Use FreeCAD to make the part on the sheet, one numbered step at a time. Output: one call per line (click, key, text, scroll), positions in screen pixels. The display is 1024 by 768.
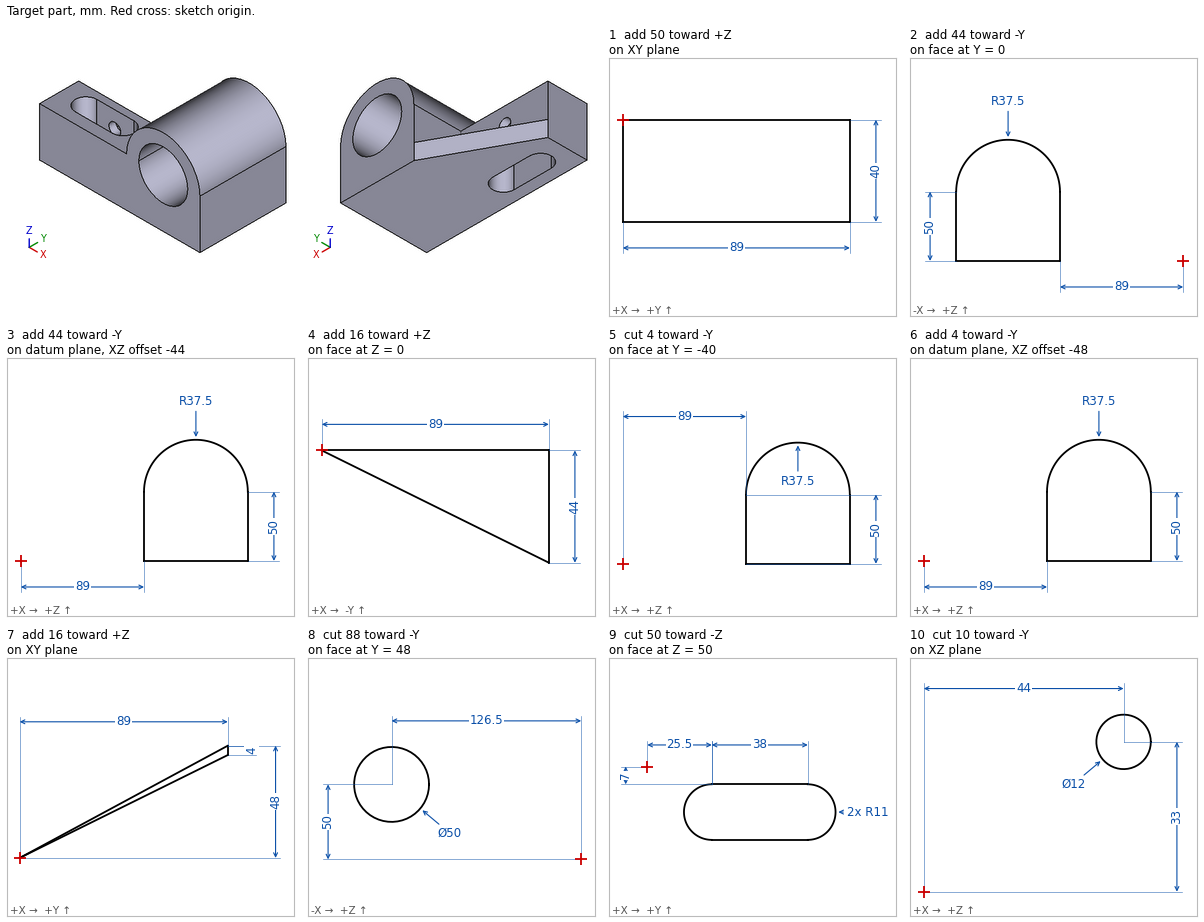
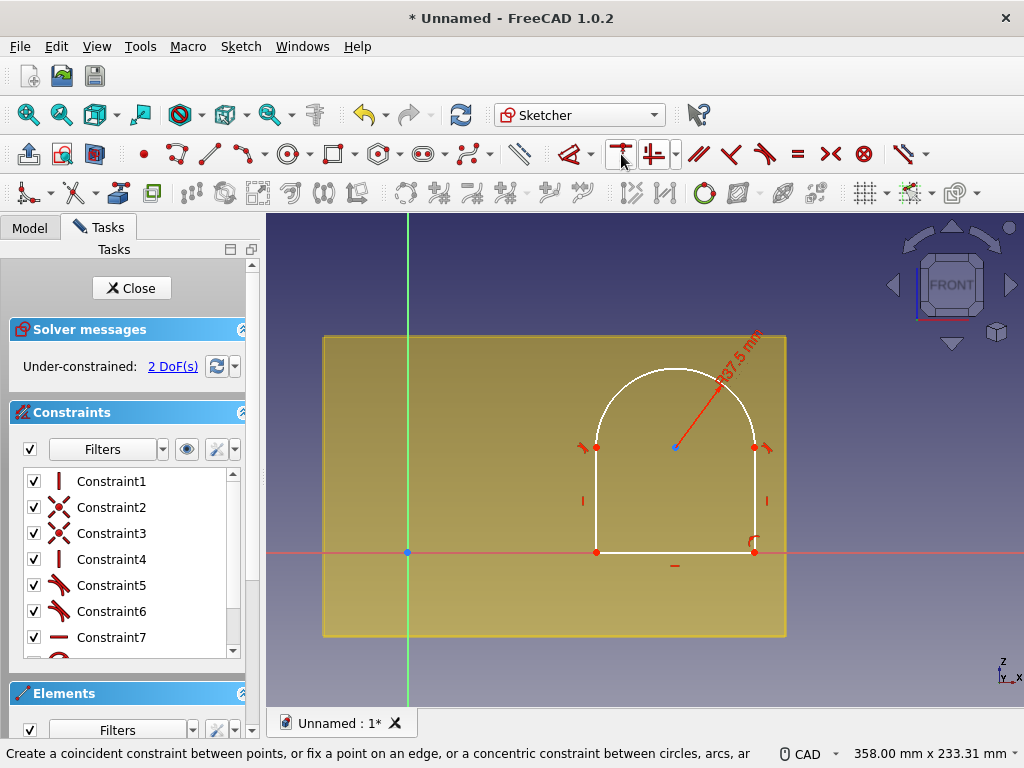
click(755, 479)
click(789, 500)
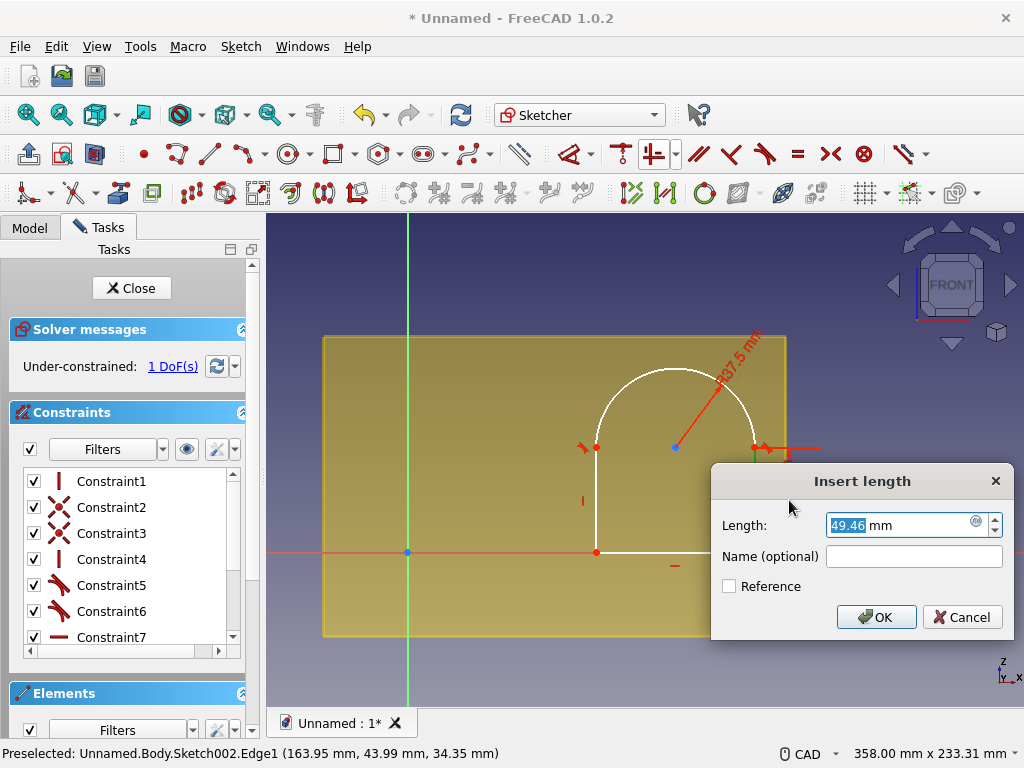
text(50)
key(Return)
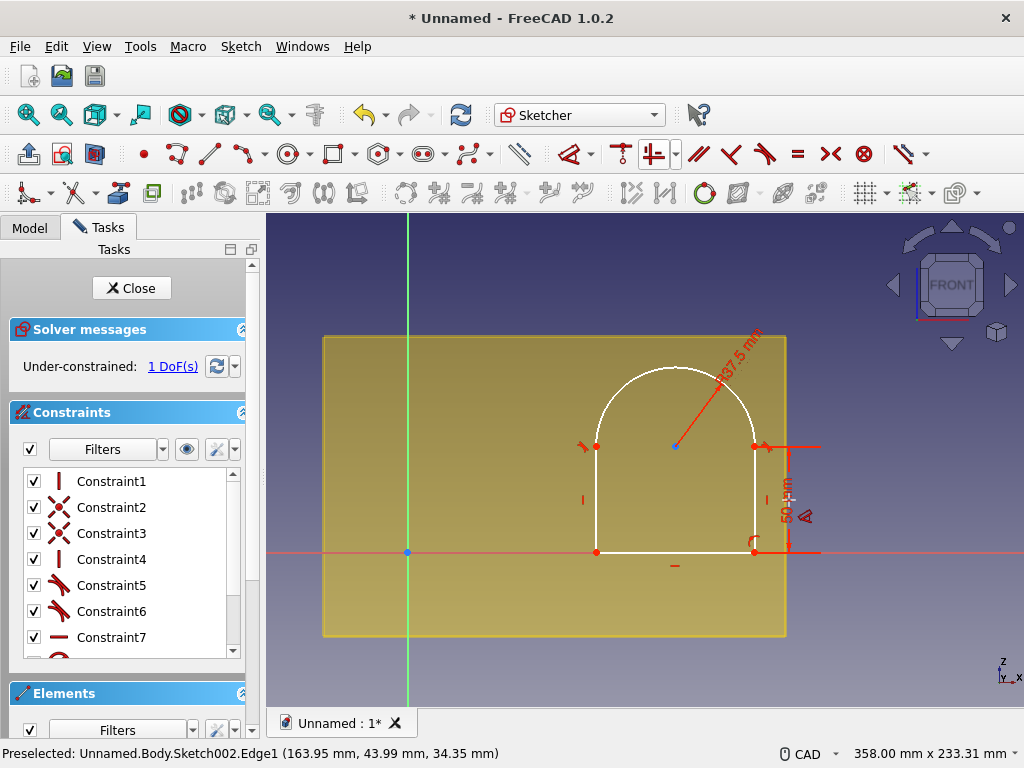
click(596, 553)
click(502, 587)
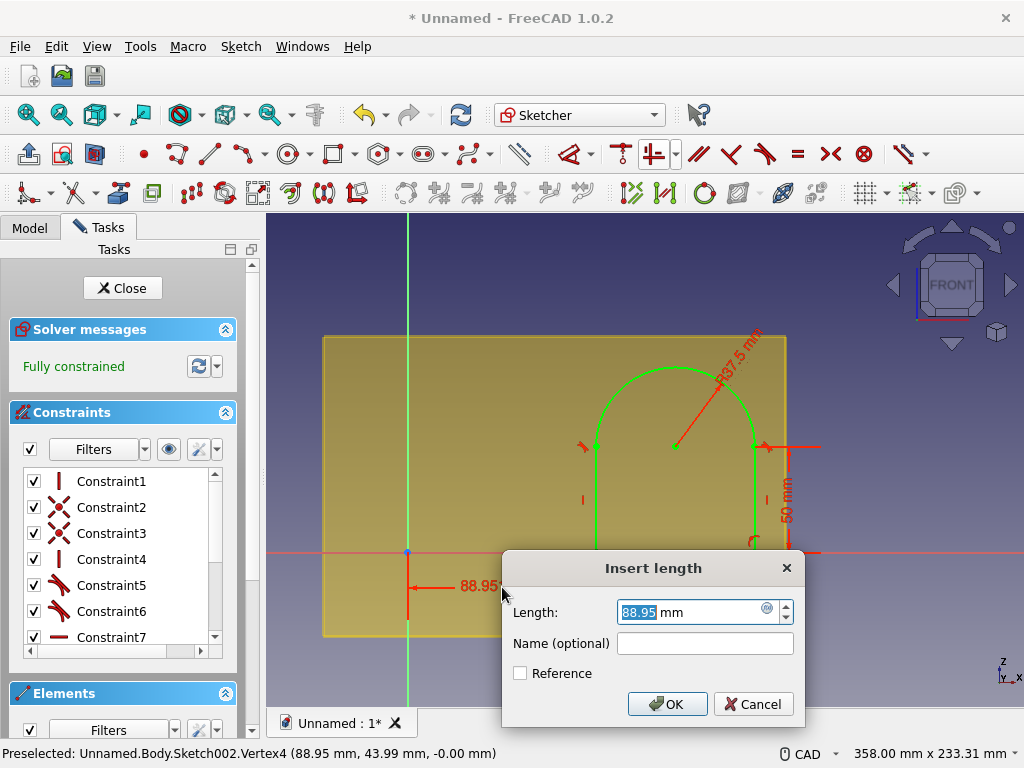
text(89)
key(Return)
key(Escape)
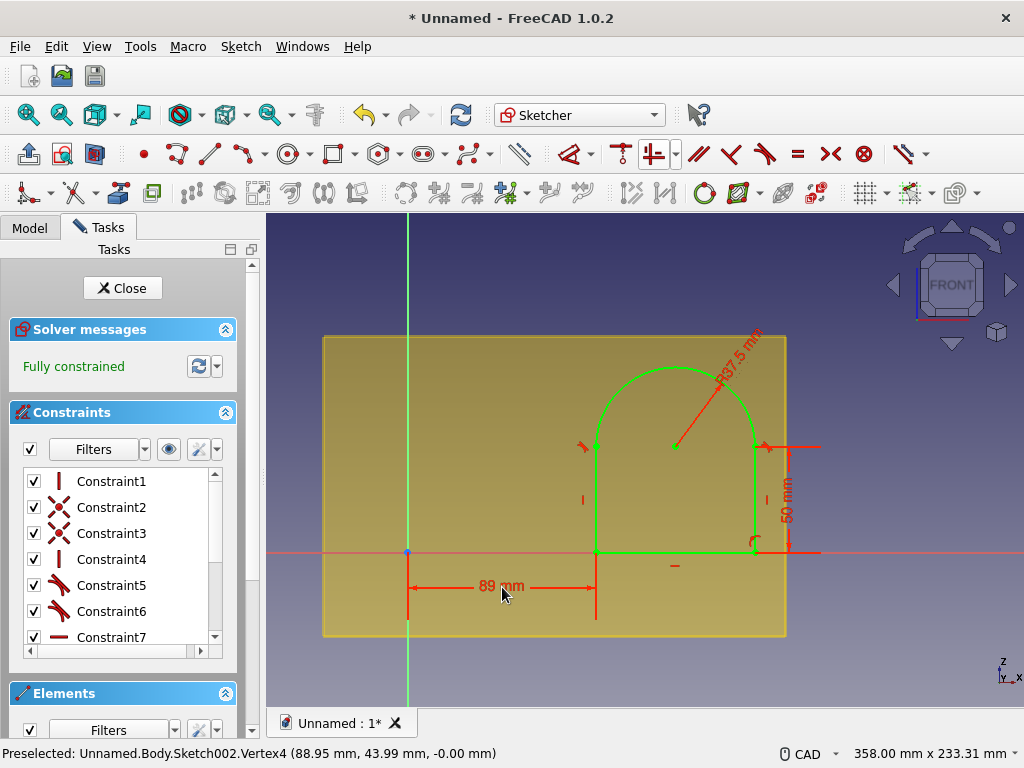
click(123, 288)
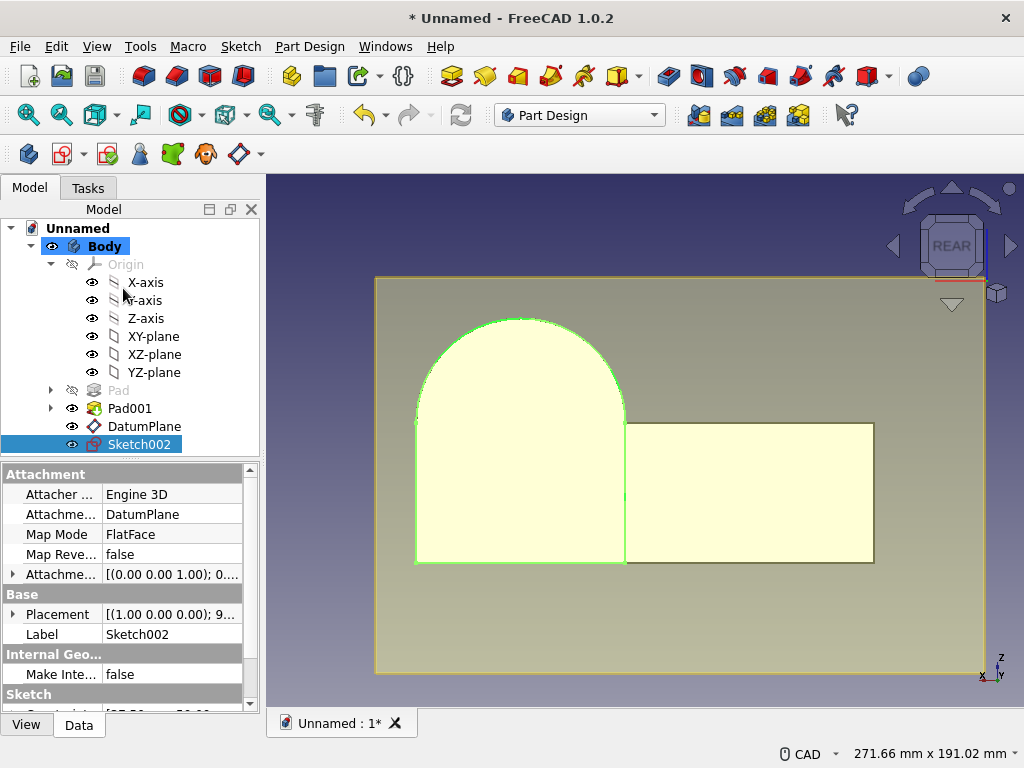
click(452, 76)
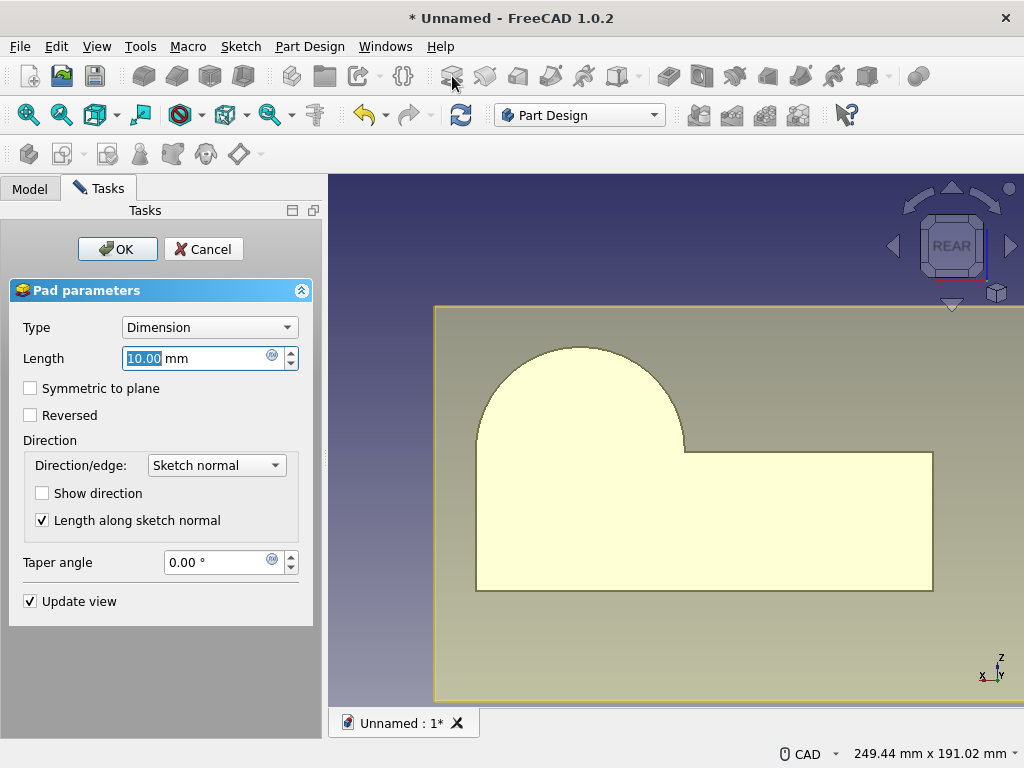
text(44)
key(Tab)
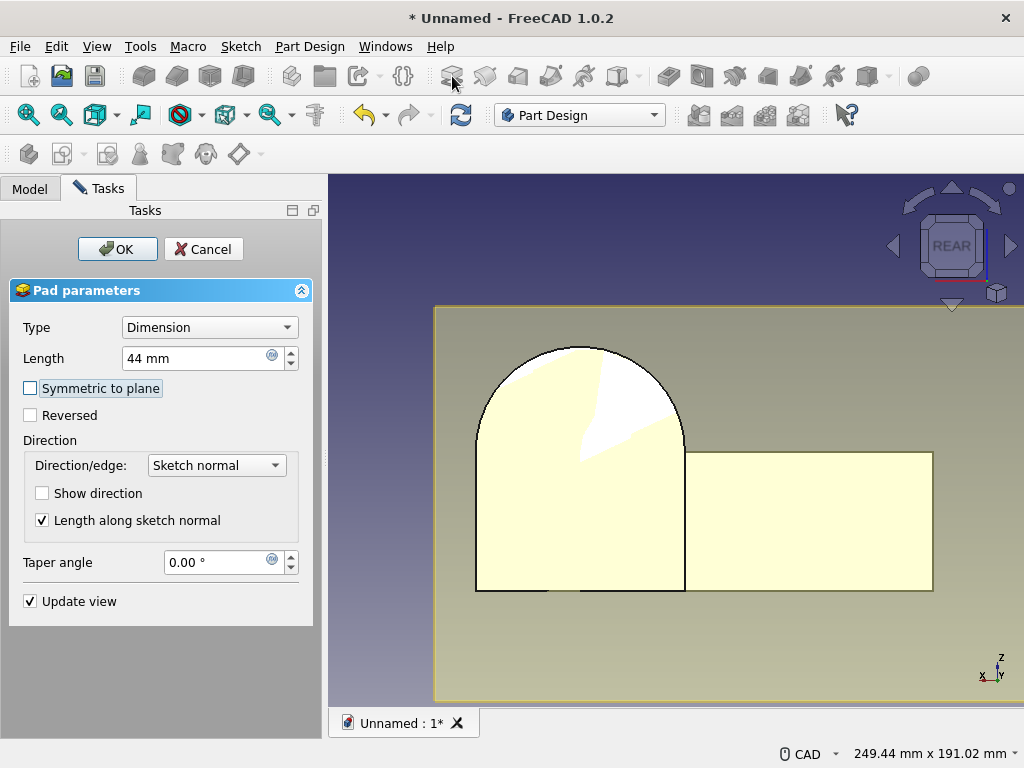
click(118, 249)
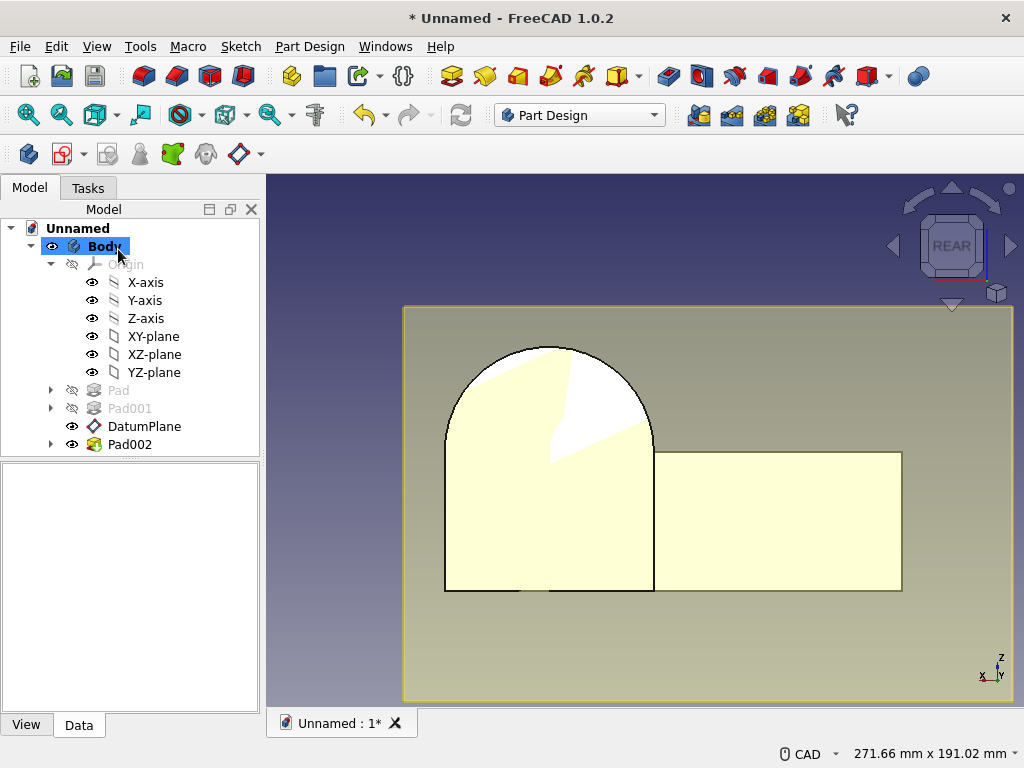
click(117, 426)
key(space)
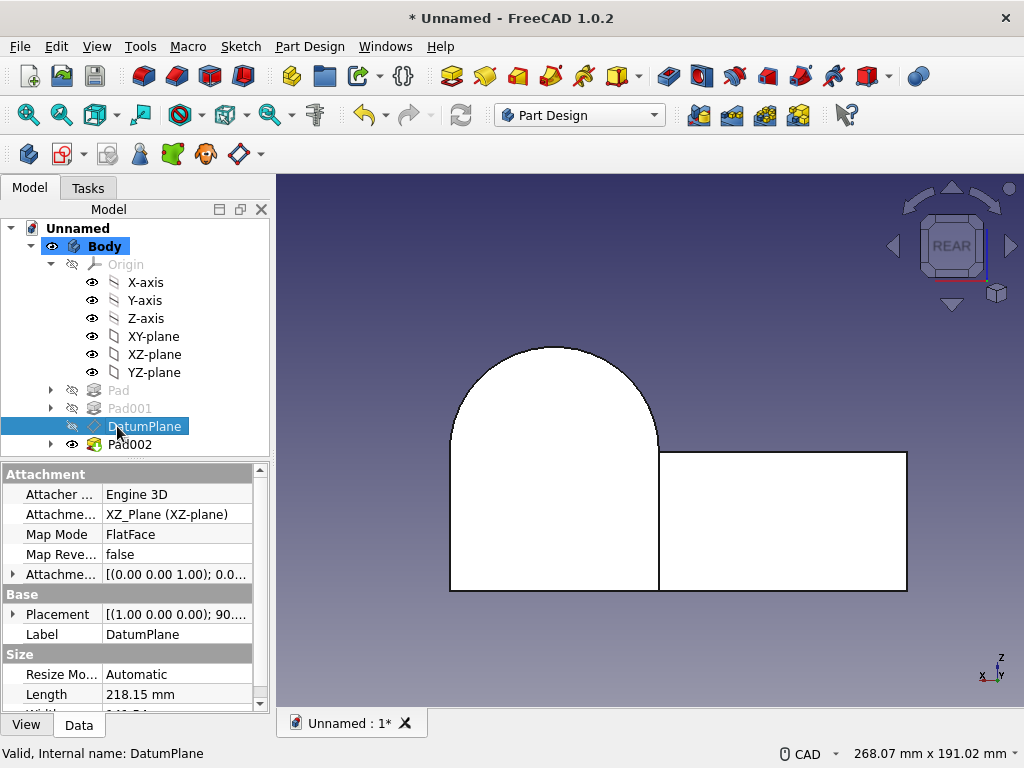
key(5)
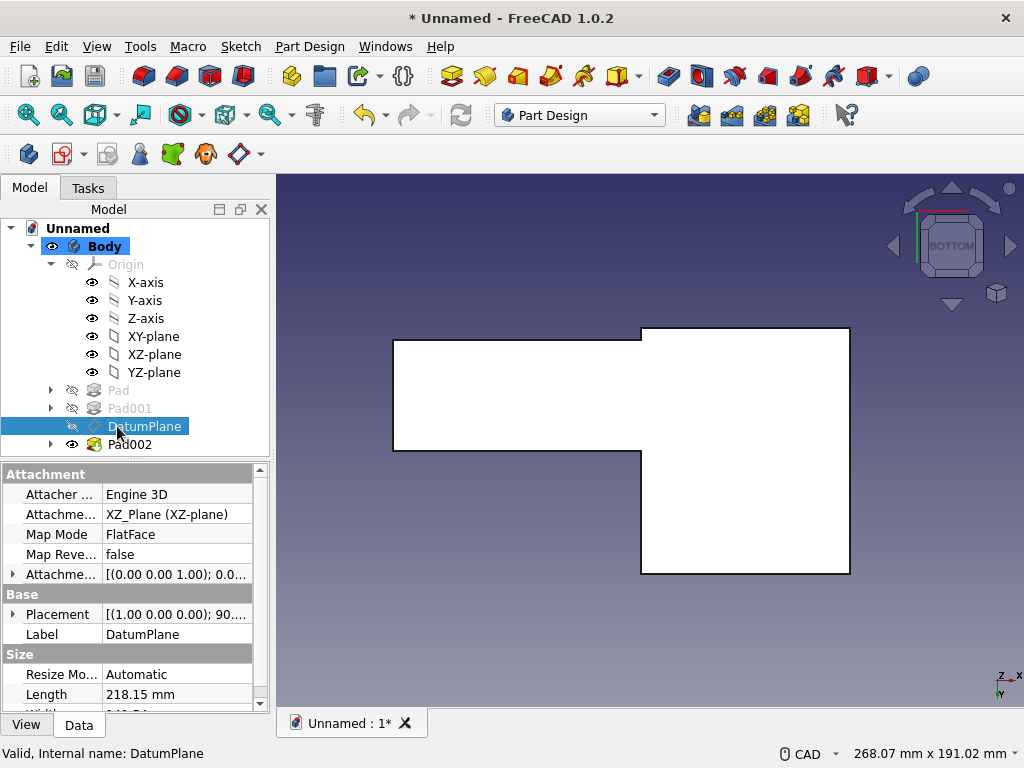
click(752, 450)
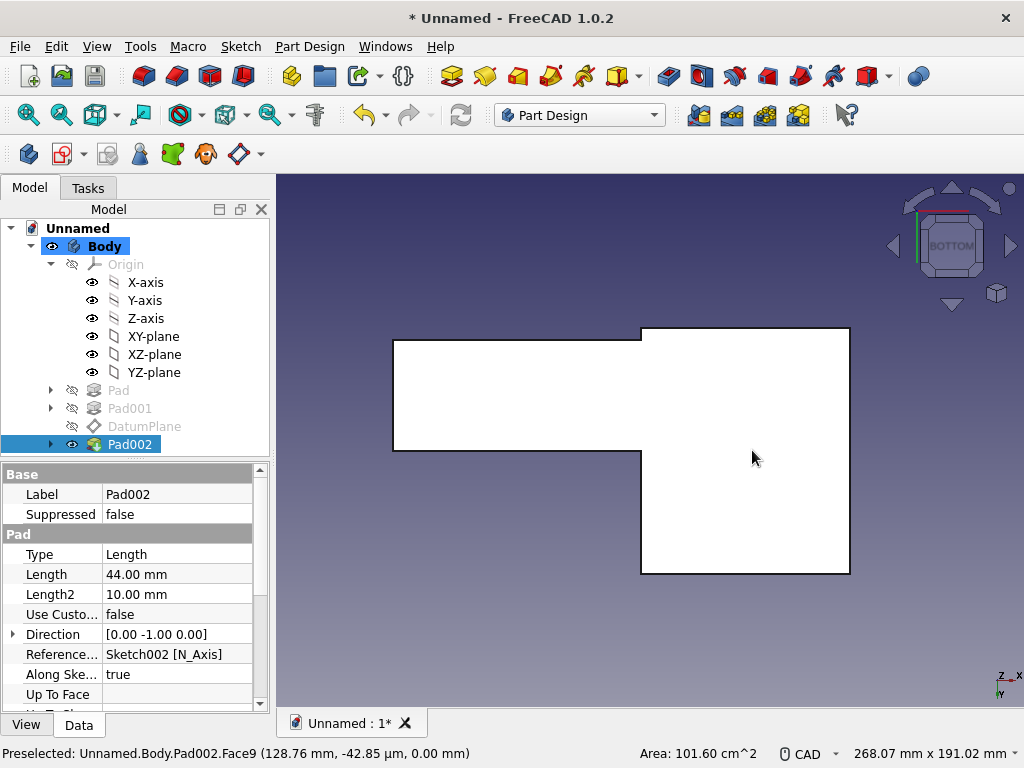
click(62, 154)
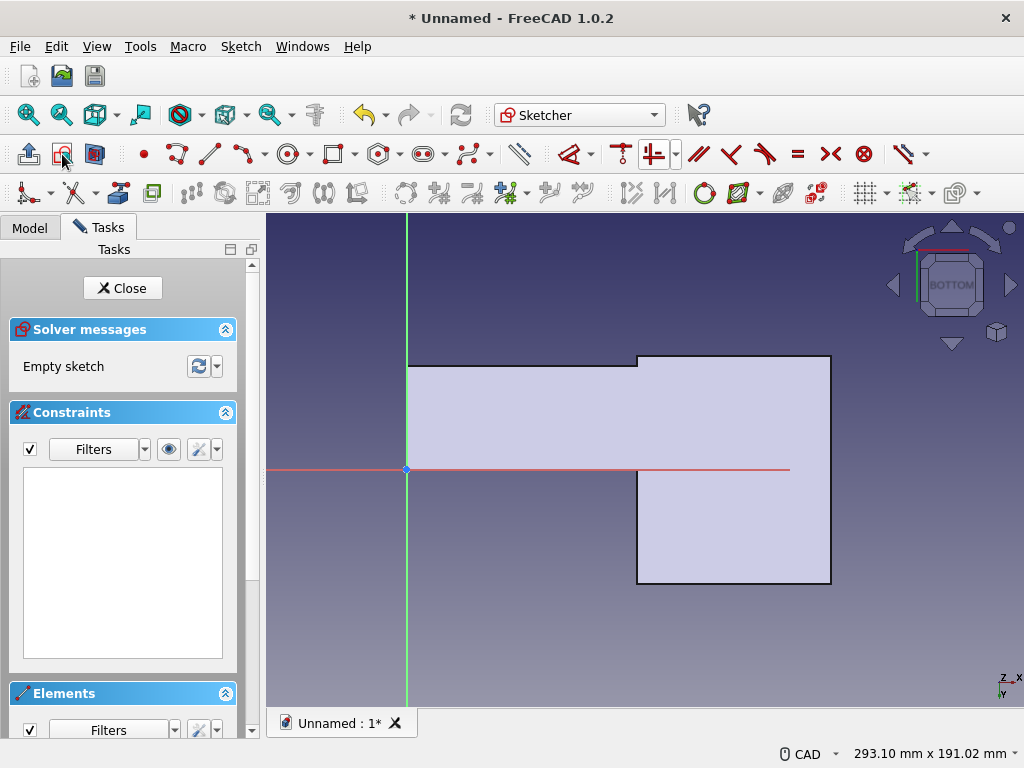
scroll(455, 608, up, 3)